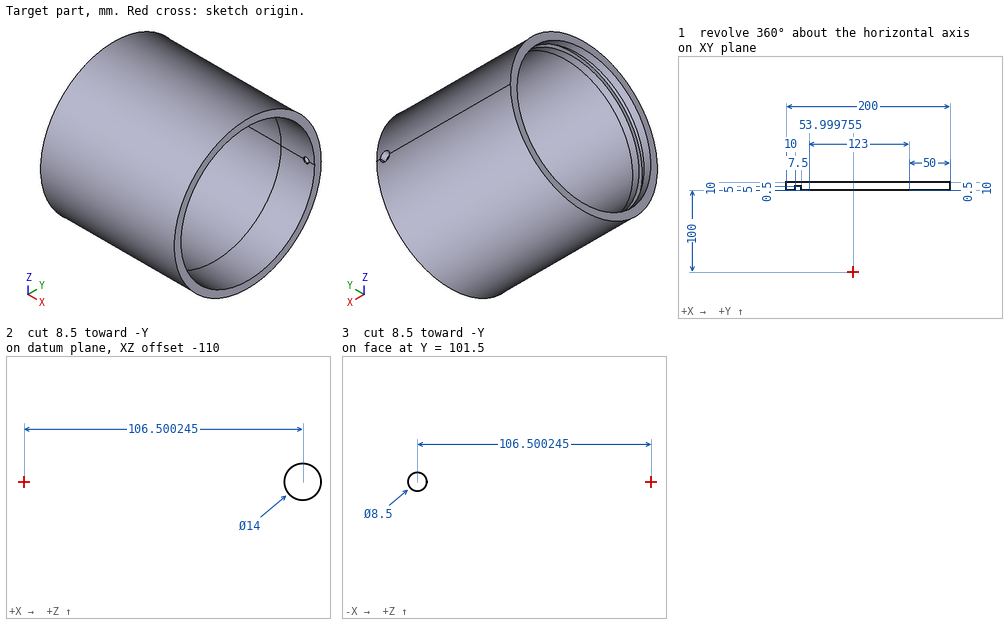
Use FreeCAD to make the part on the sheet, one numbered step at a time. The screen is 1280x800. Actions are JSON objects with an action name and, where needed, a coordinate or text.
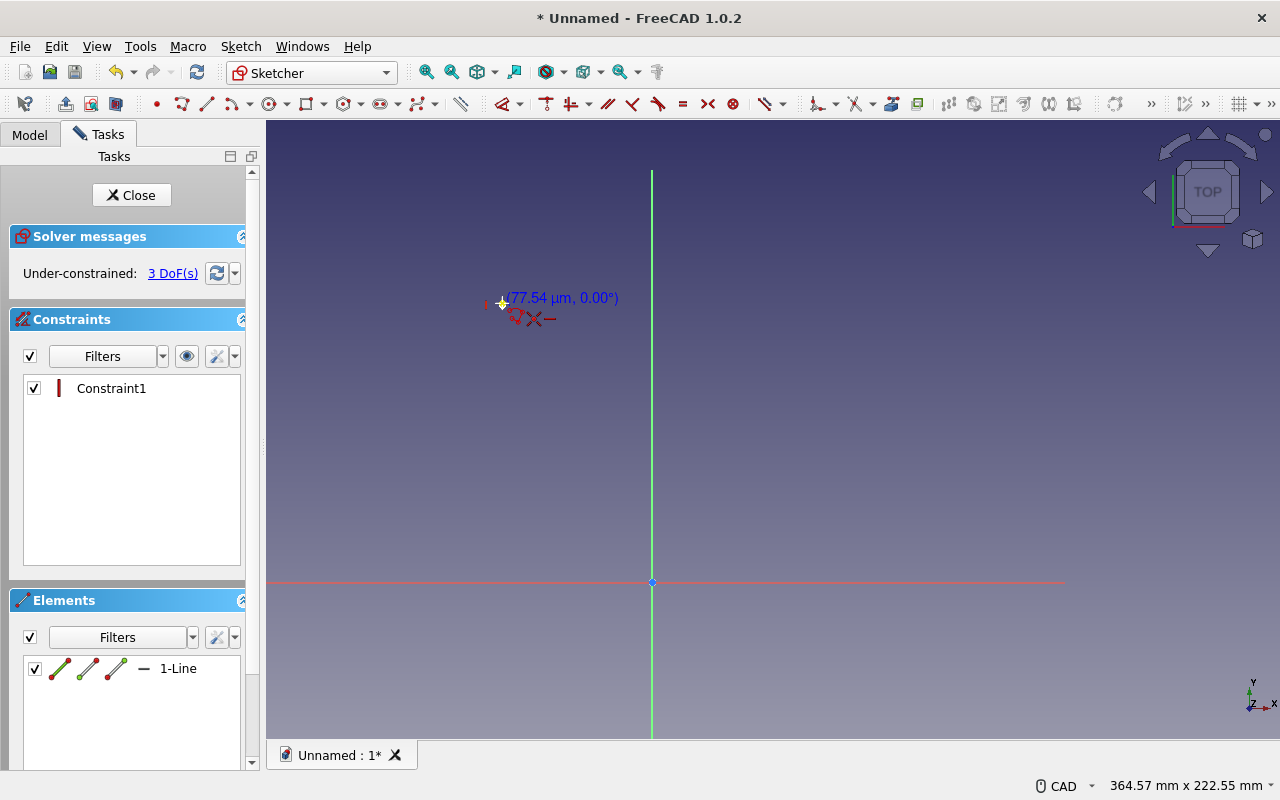
{"action": "left_click", "coordinate": [844, 303]}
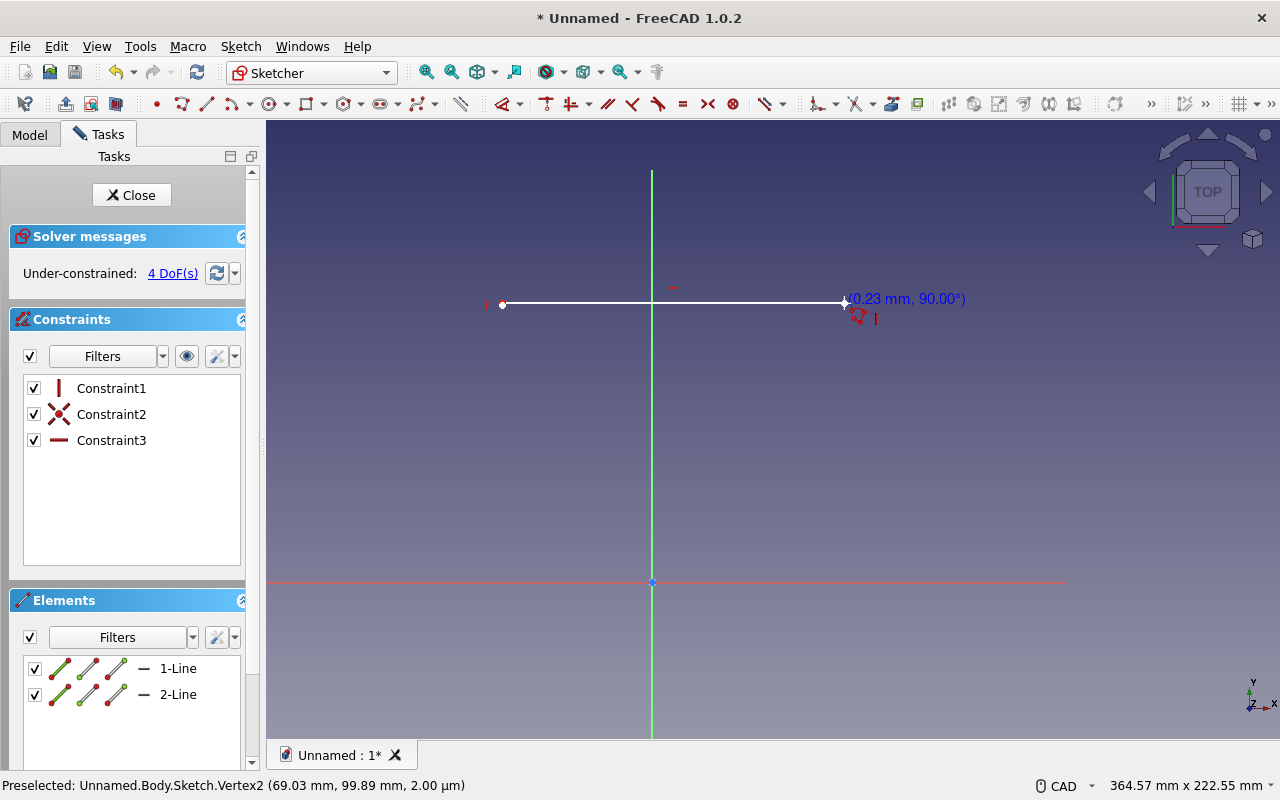
{"action": "scroll", "coordinate": [844, 305], "scroll_direction": "up", "scroll_amount": 13}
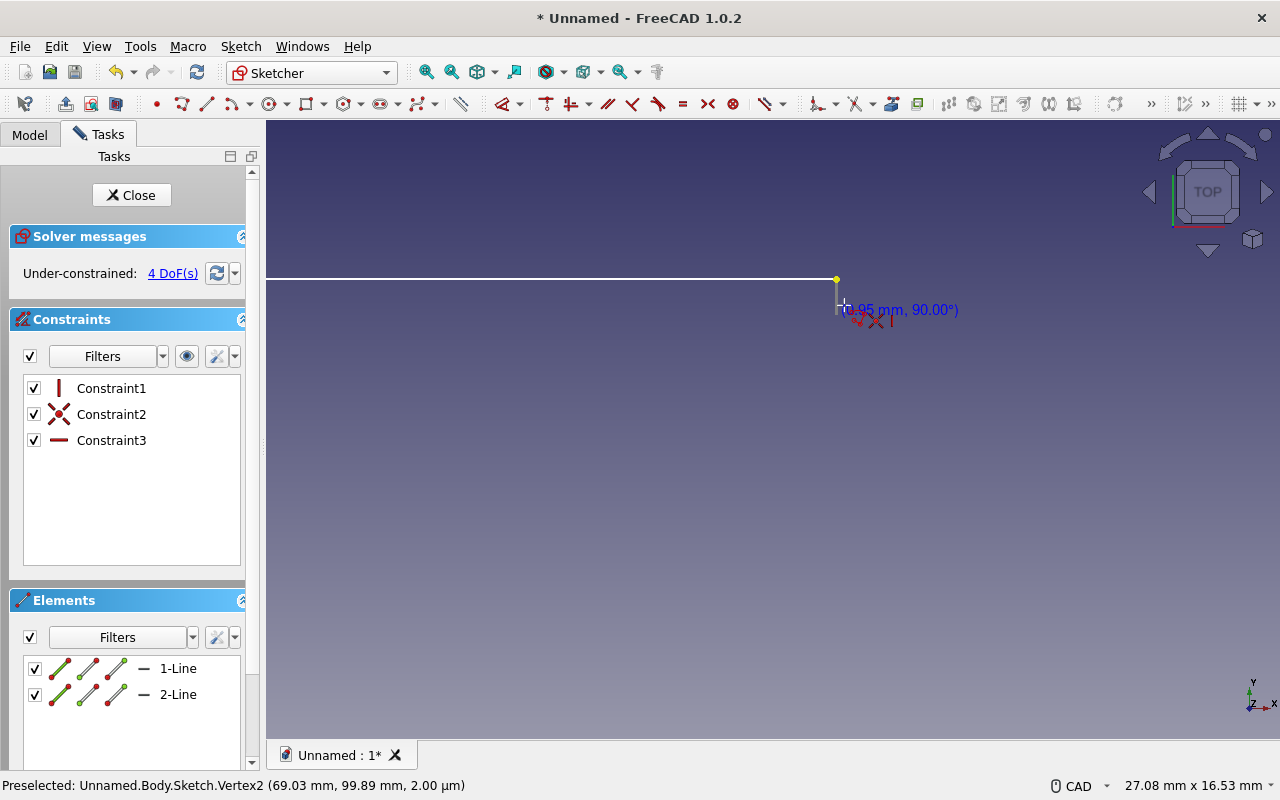
{"action": "left_click", "coordinate": [837, 297]}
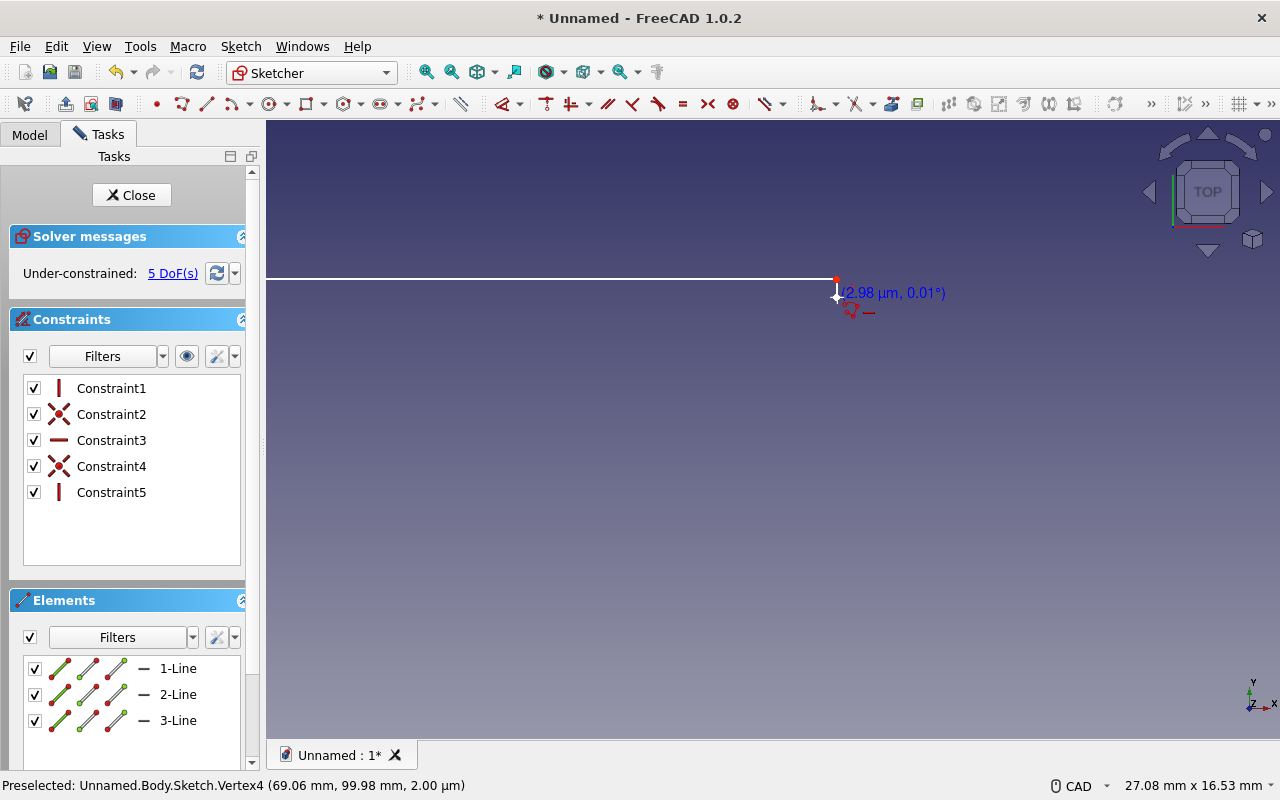
{"action": "scroll", "coordinate": [844, 305], "scroll_direction": "down", "scroll_amount": 13}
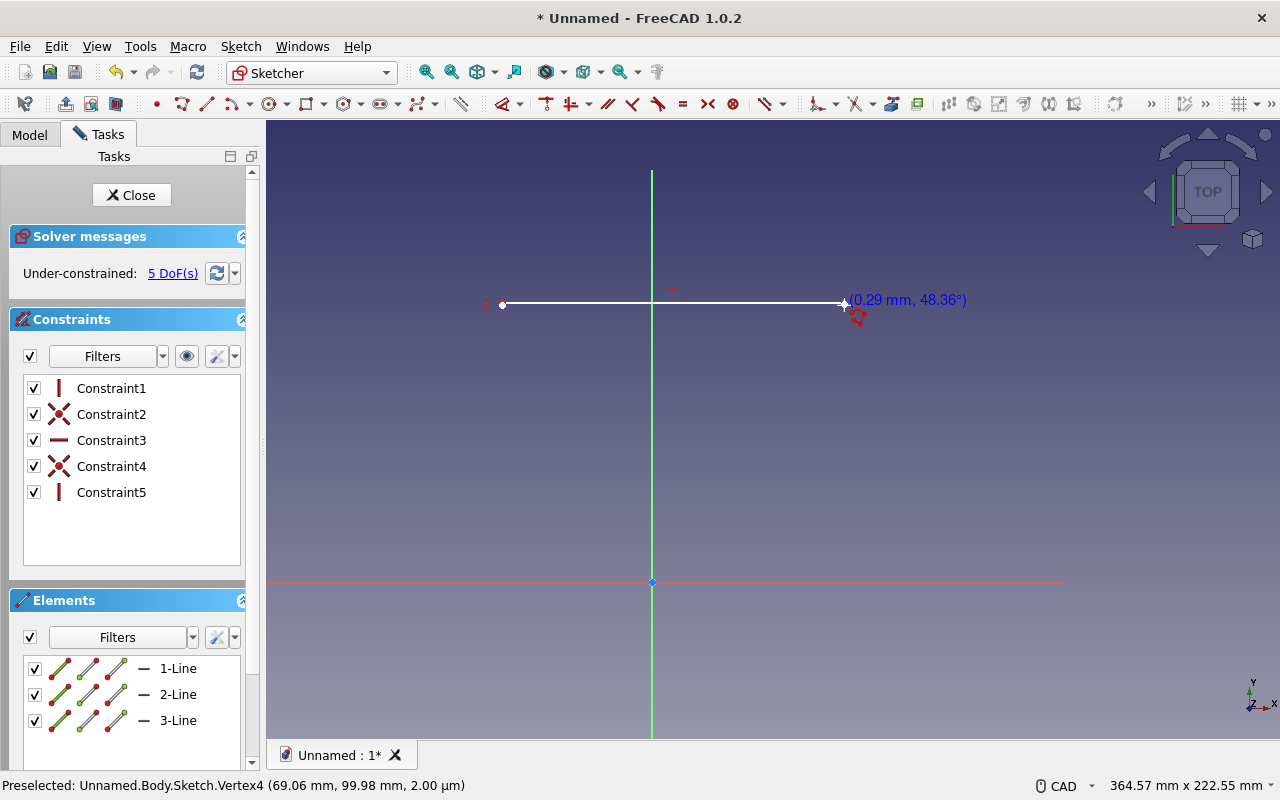
{"action": "left_click", "coordinate": [983, 305]}
{"action": "left_click", "coordinate": [983, 277]}
{"action": "left_click", "coordinate": [427, 277]}
{"action": "left_click", "coordinate": [427, 305]}
{"action": "left_click", "coordinate": [455, 305]}
{"action": "left_click", "coordinate": [455, 291]}
{"action": "left_click", "coordinate": [475, 291]}
{"action": "left_click", "coordinate": [475, 305]}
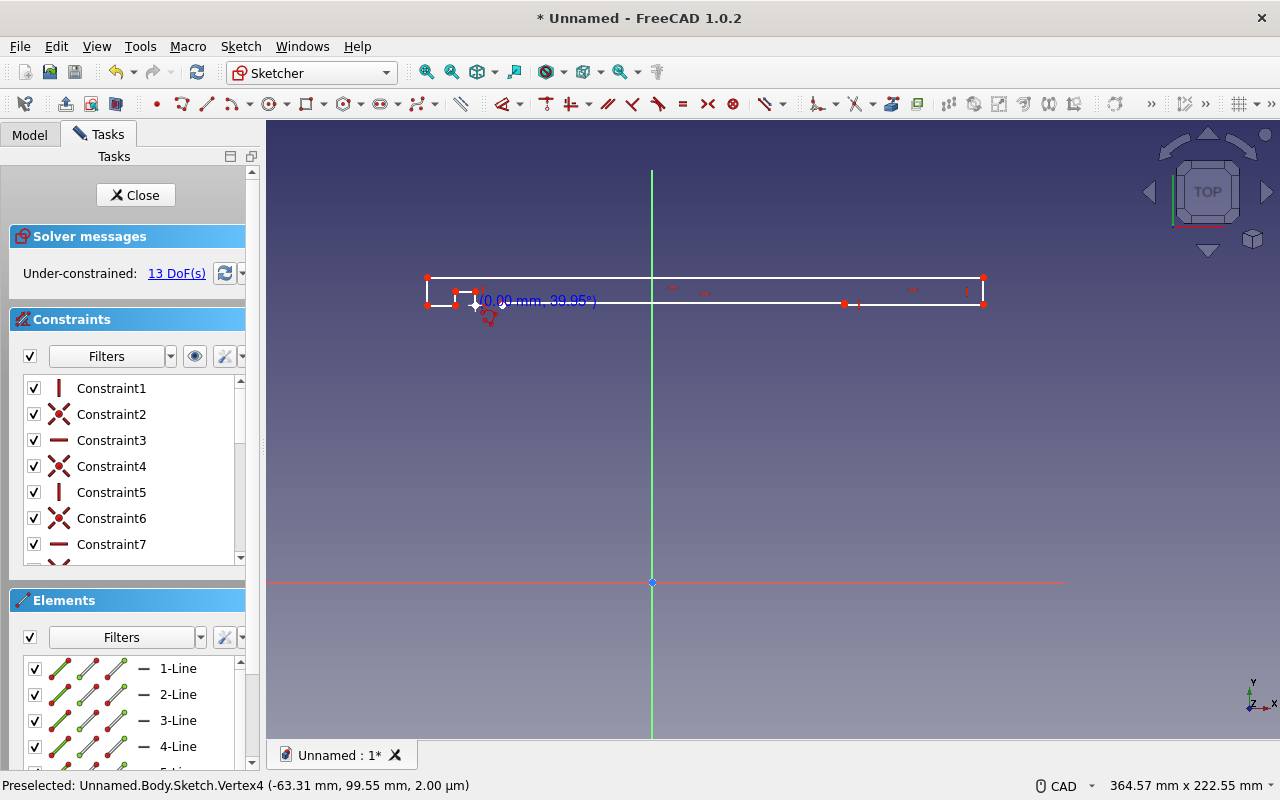
{"action": "scroll", "coordinate": [502, 305], "scroll_direction": "up", "scroll_amount": 16}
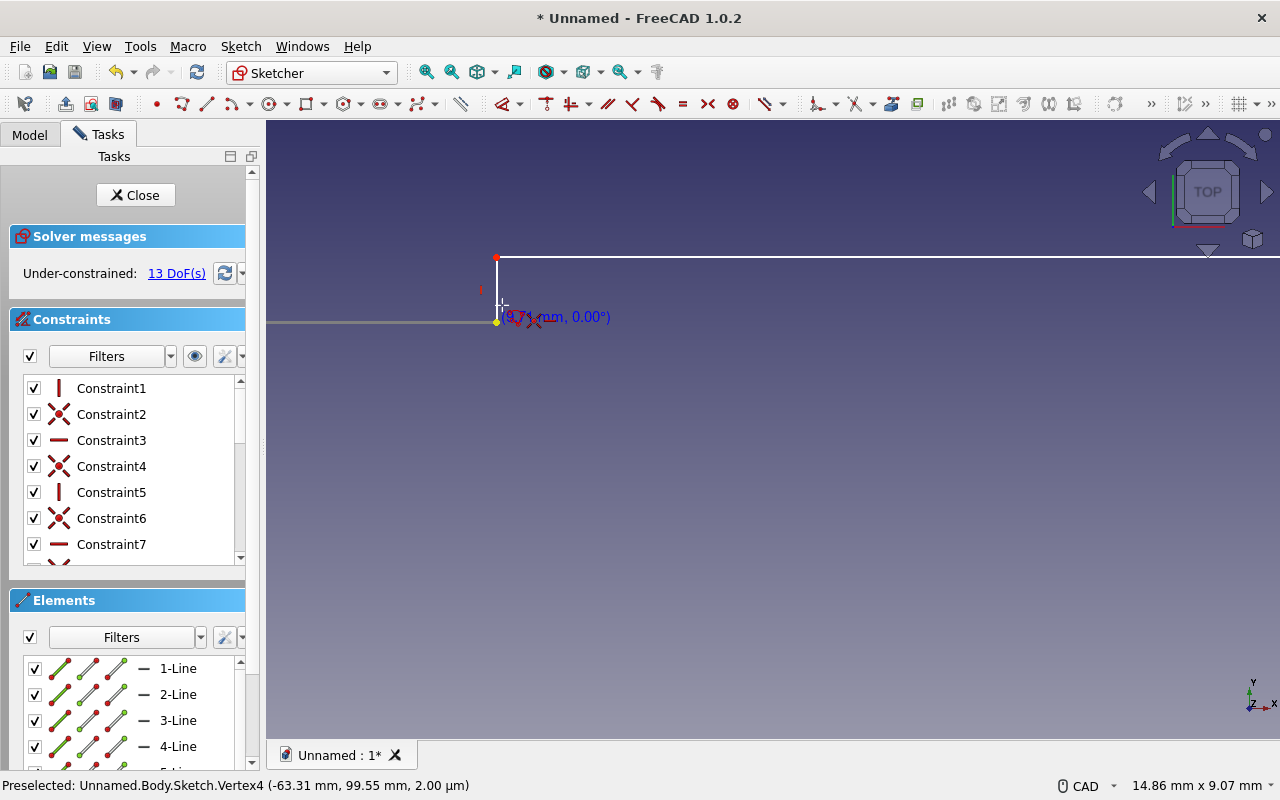
{"action": "left_click", "coordinate": [497, 298]}
{"action": "key", "text": "Escape"}
{"action": "key", "text": "Escape"}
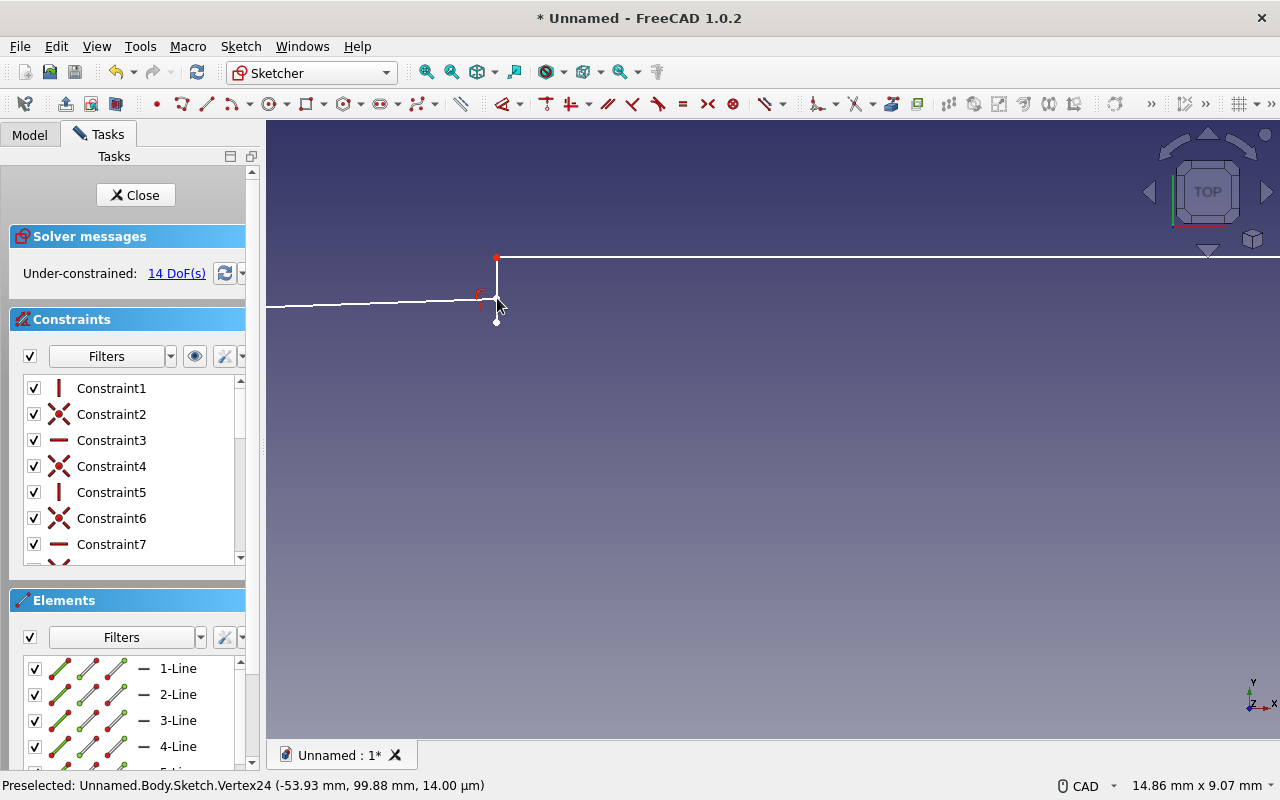
{"action": "scroll", "coordinate": [455, 276], "scroll_direction": "down", "scroll_amount": 15}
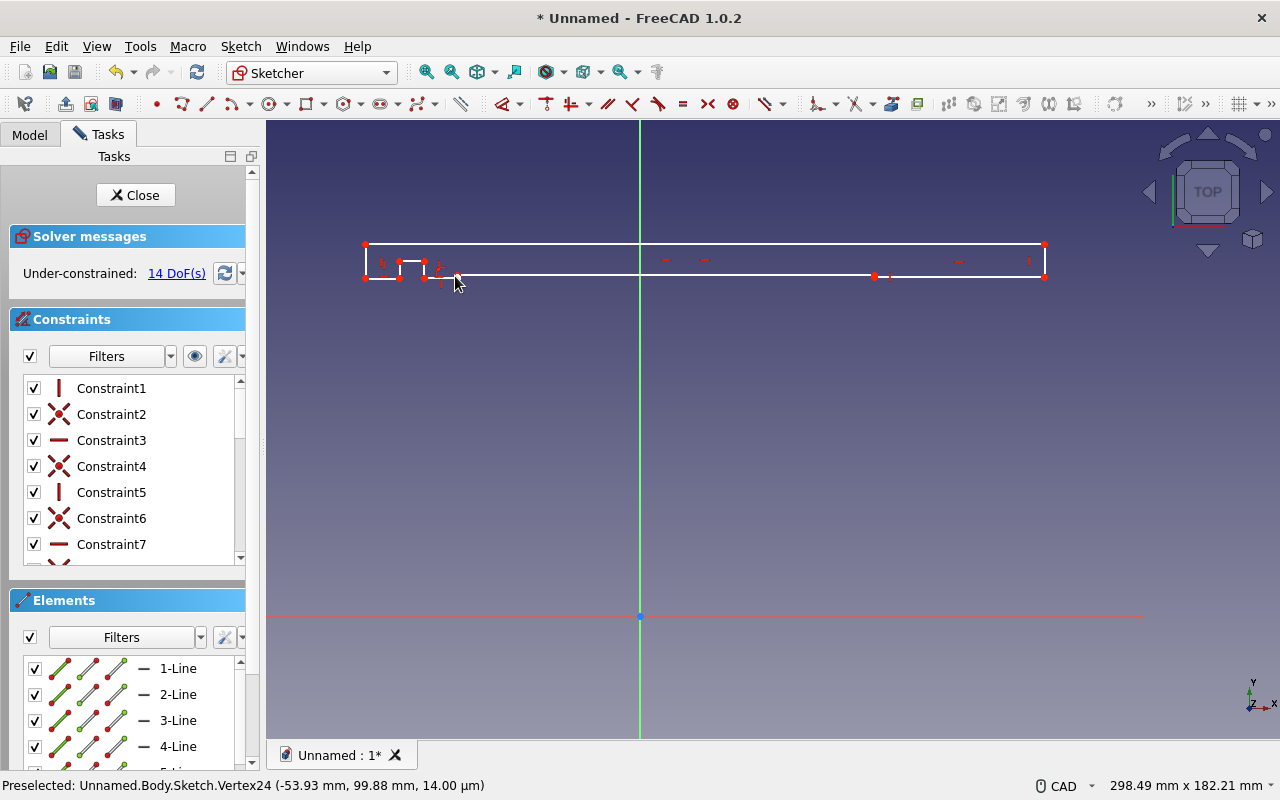
{"action": "scroll", "coordinate": [447, 278], "scroll_direction": "up", "scroll_amount": 2}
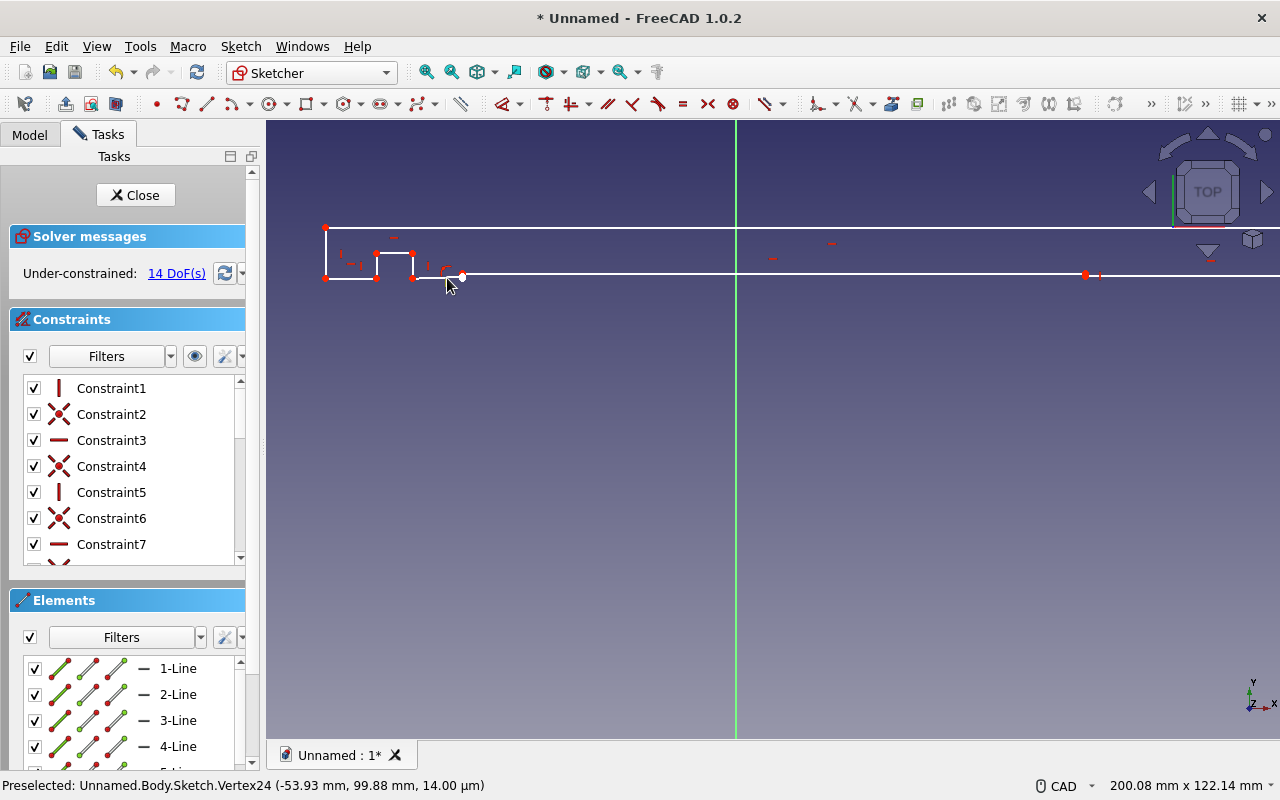
{"action": "left_click", "coordinate": [428, 278]}